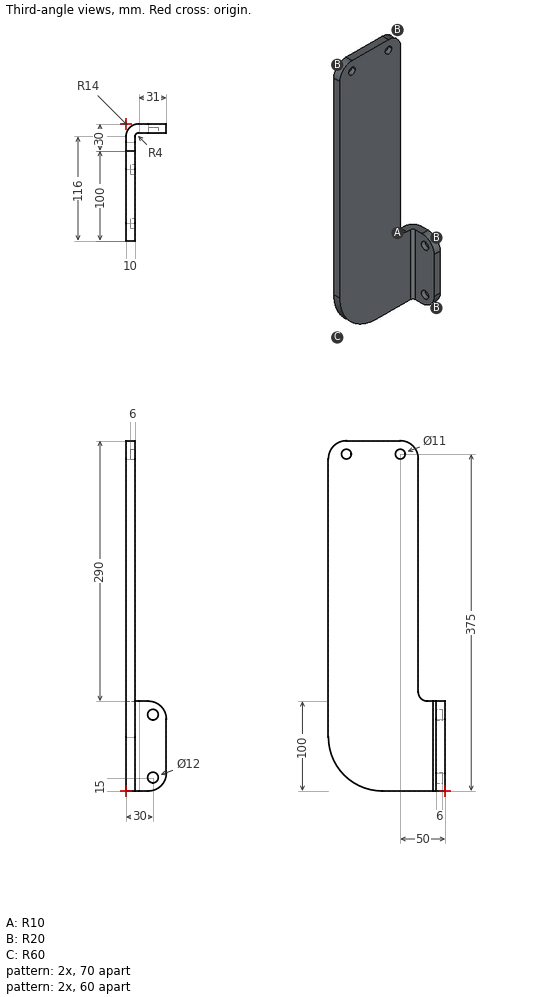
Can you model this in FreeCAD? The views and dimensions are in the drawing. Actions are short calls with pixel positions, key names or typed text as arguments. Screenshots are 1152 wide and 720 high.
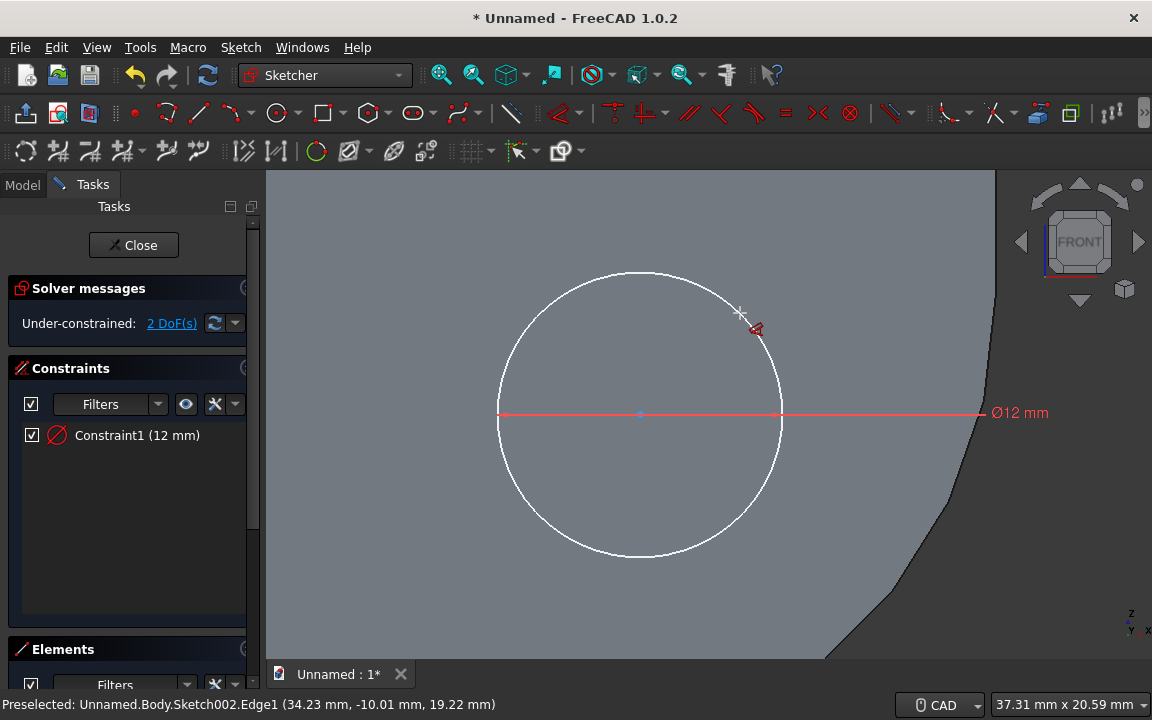
click(640, 415)
click(467, 381)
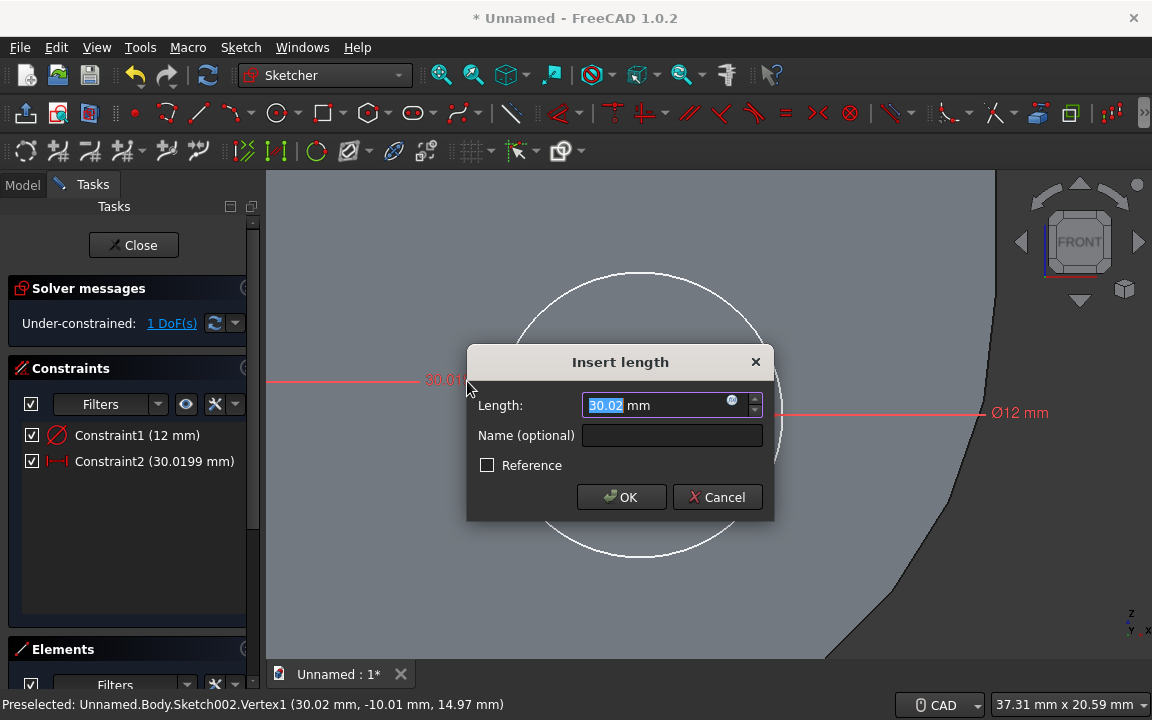
text(30)
key(Return)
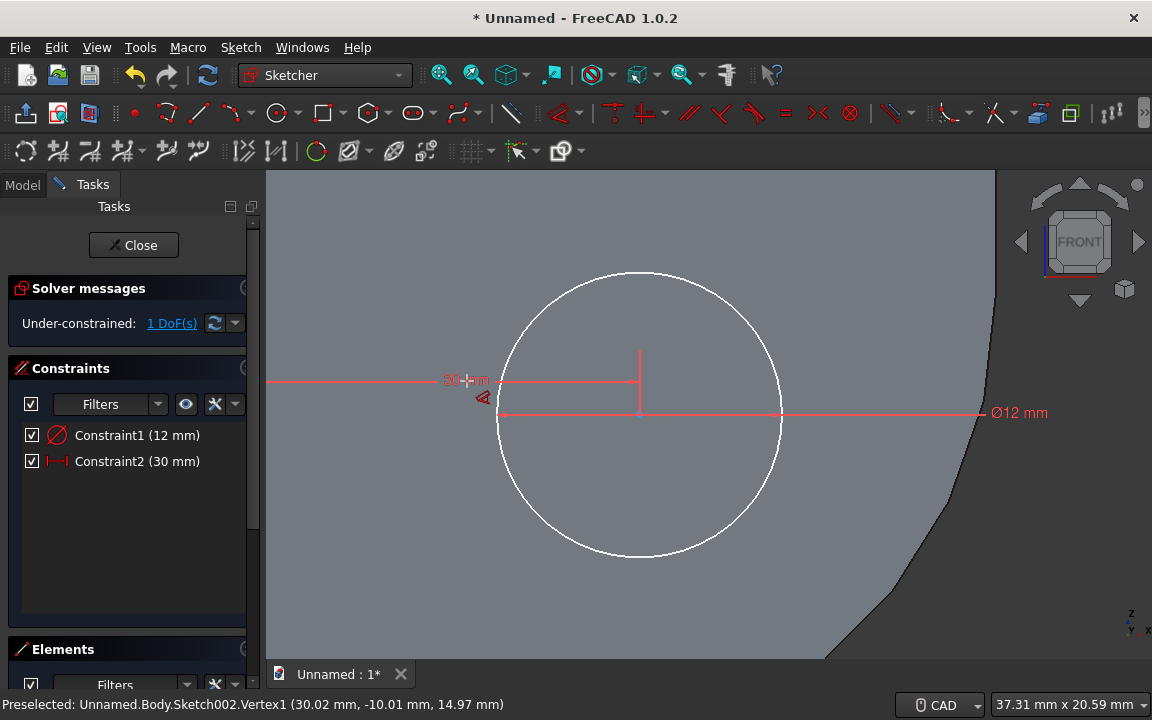
click(640, 415)
click(674, 523)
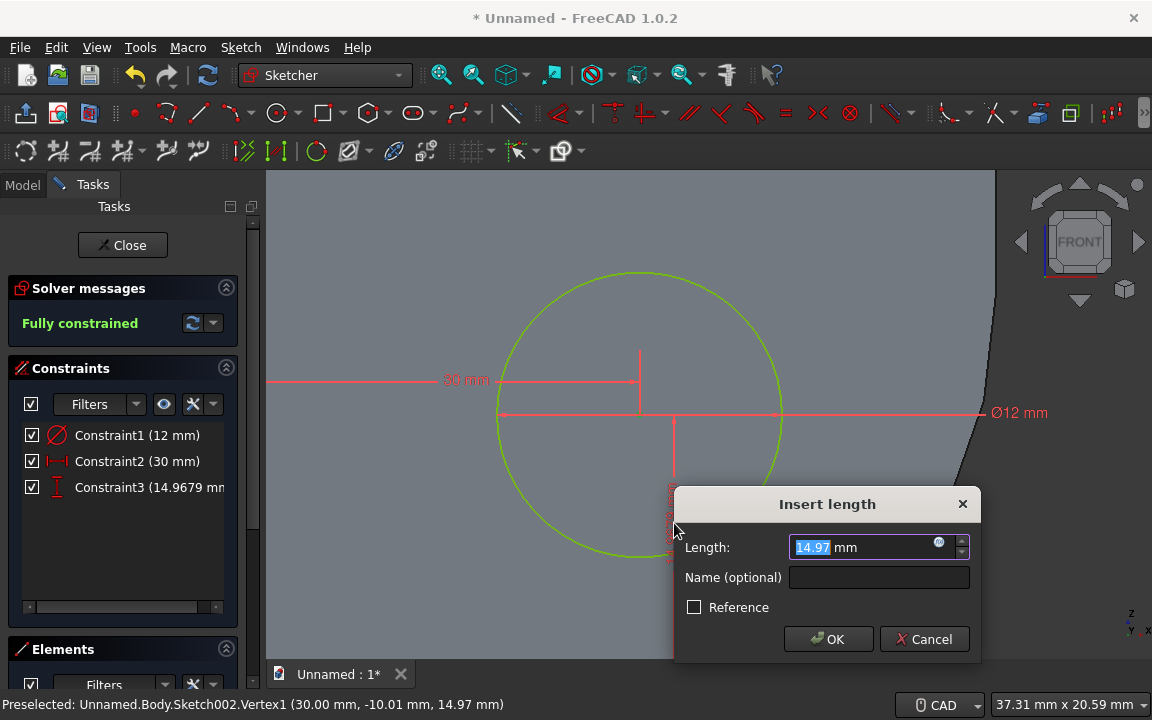
text(15)
key(Return)
key(Escape)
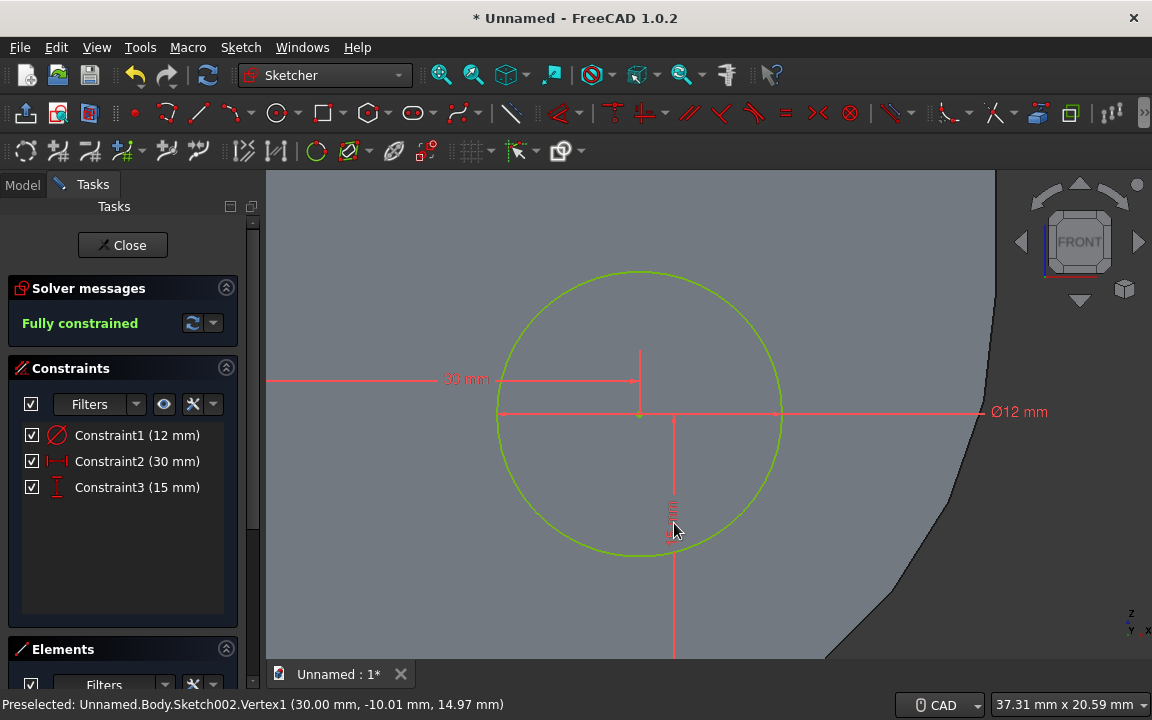
click(123, 245)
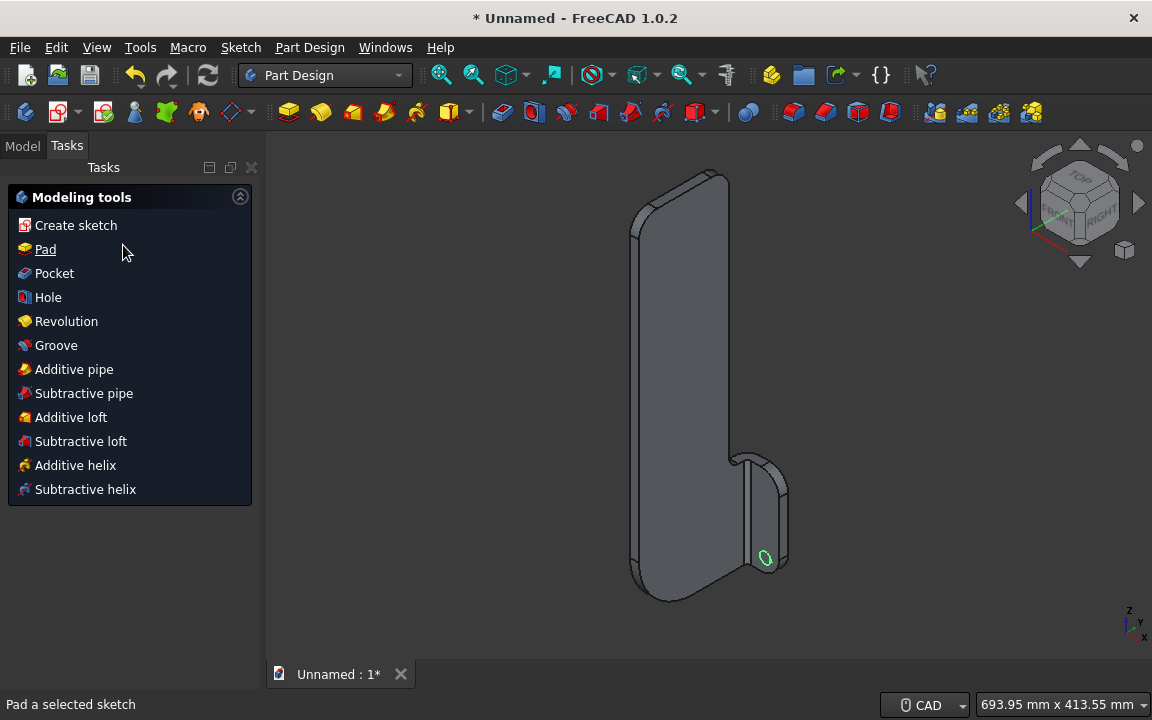
click(504, 112)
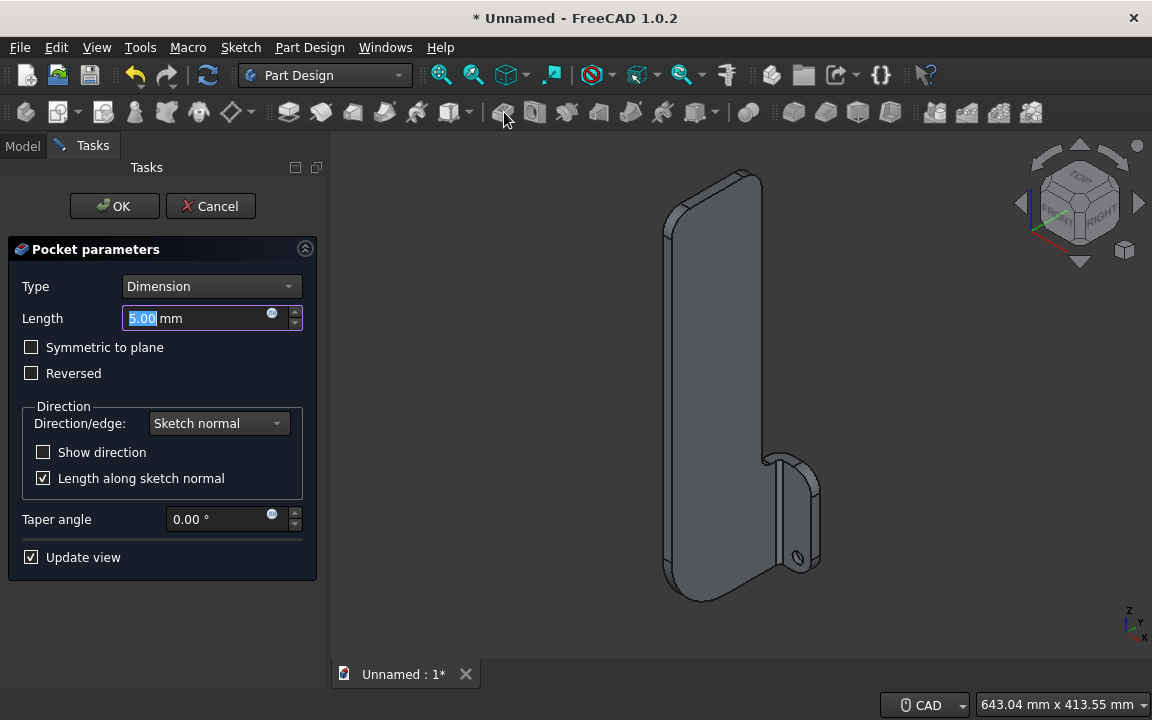
text(6)
key(Tab)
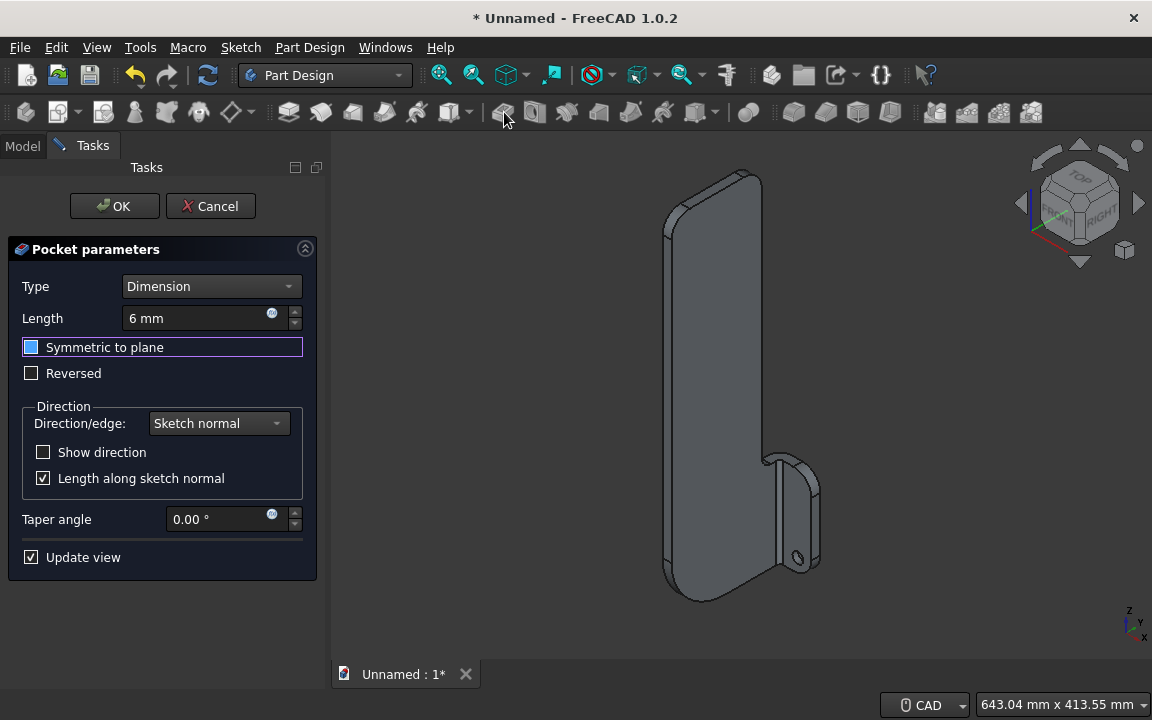
click(115, 206)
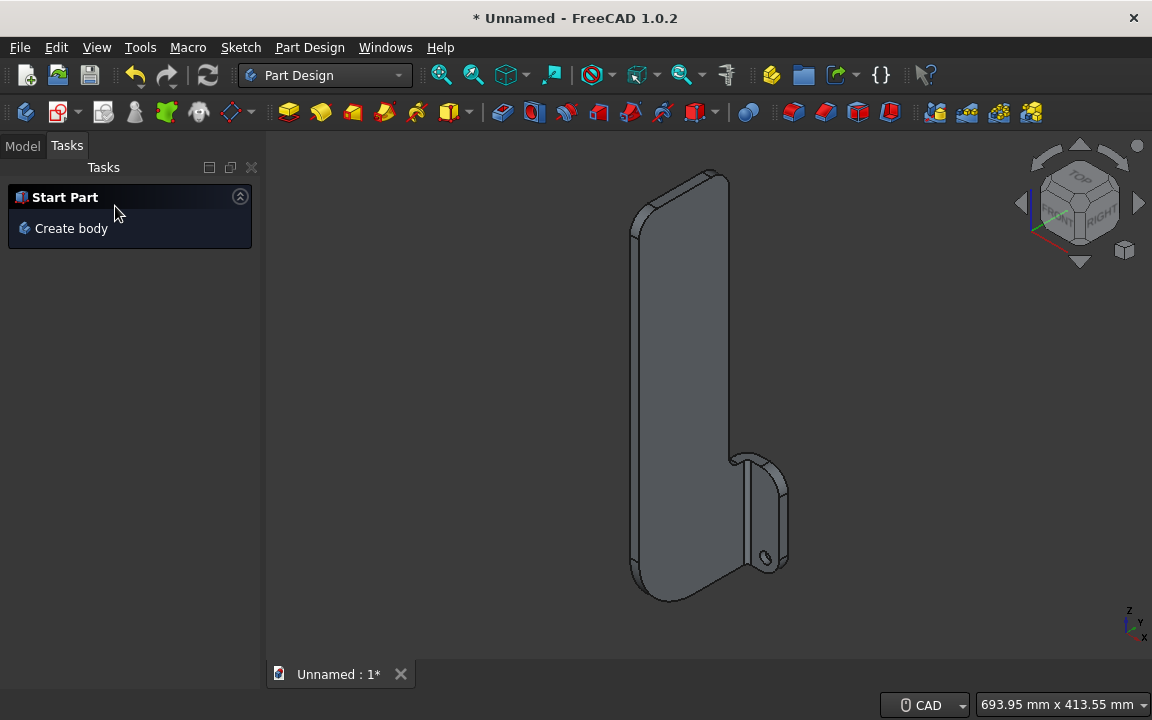
click(23, 145)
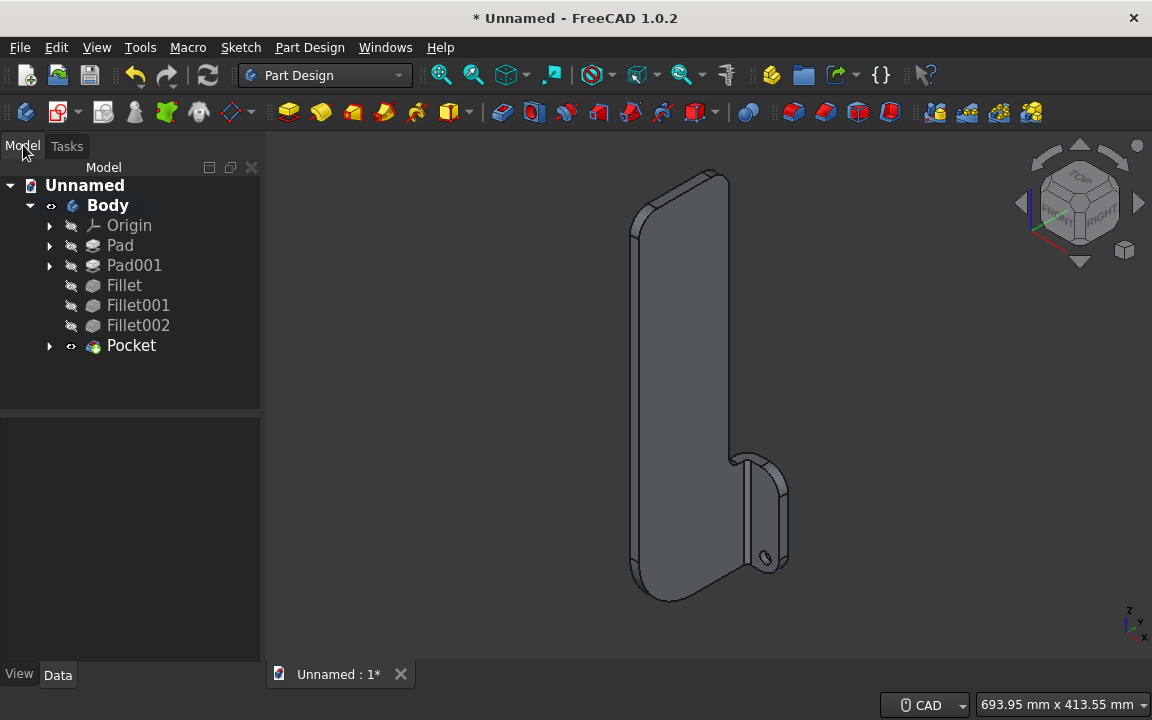
click(116, 346)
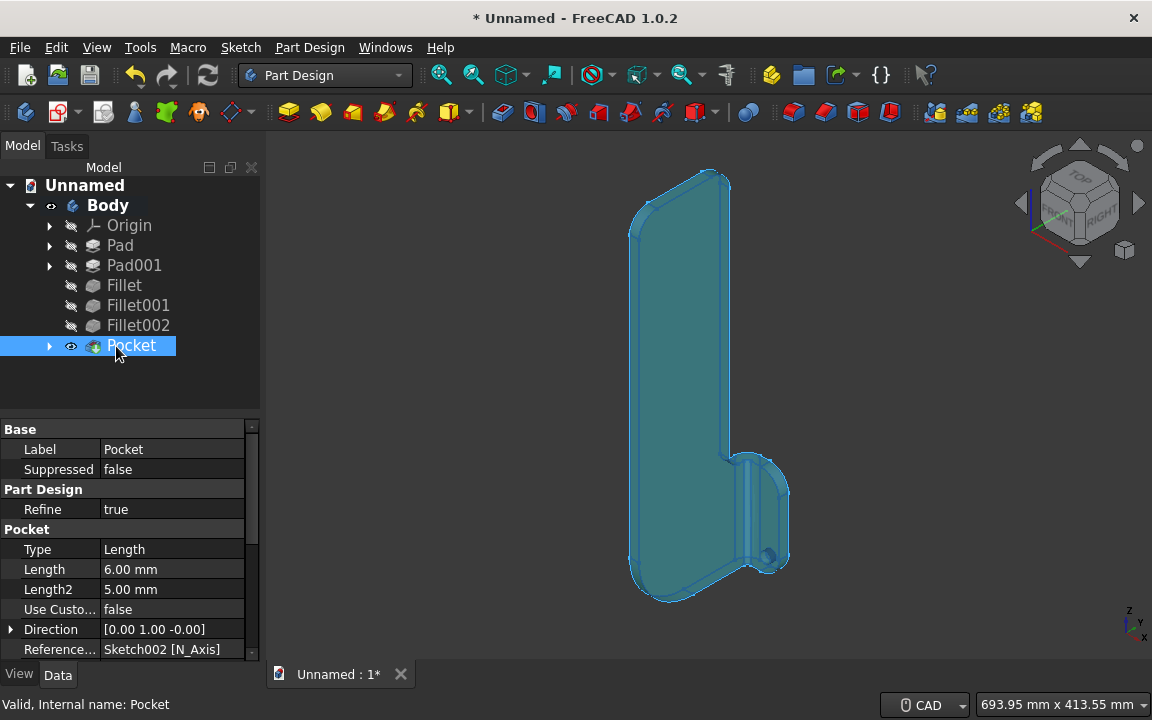
click(968, 112)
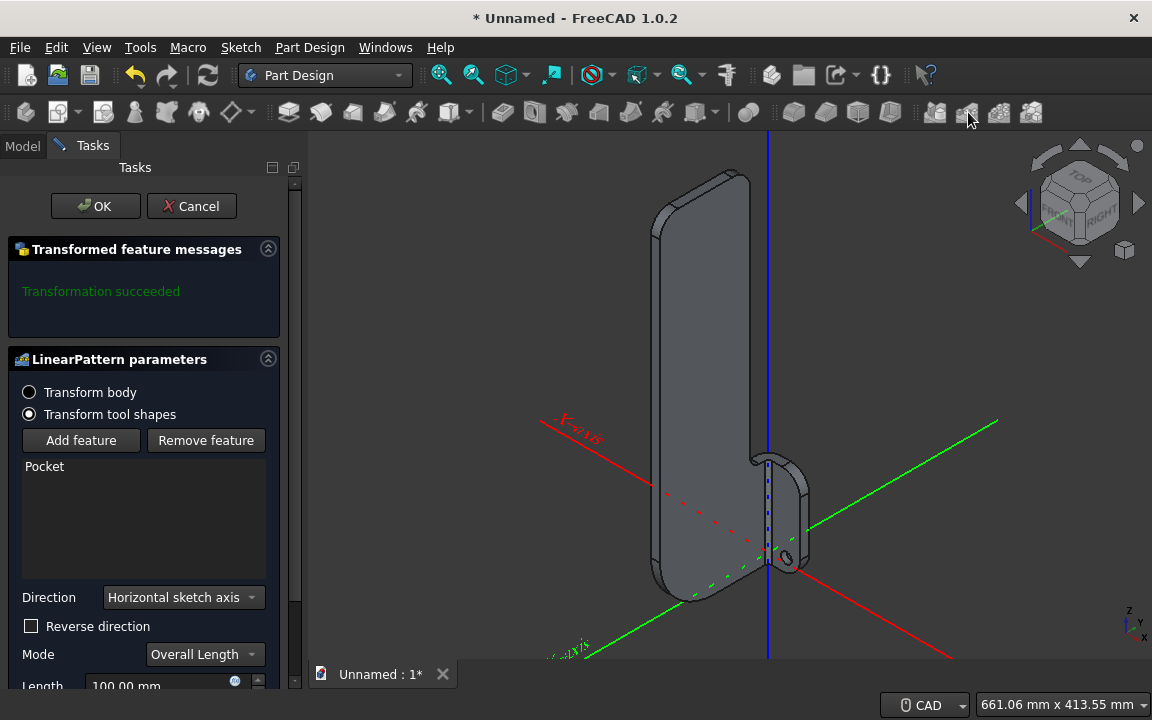
click(184, 598)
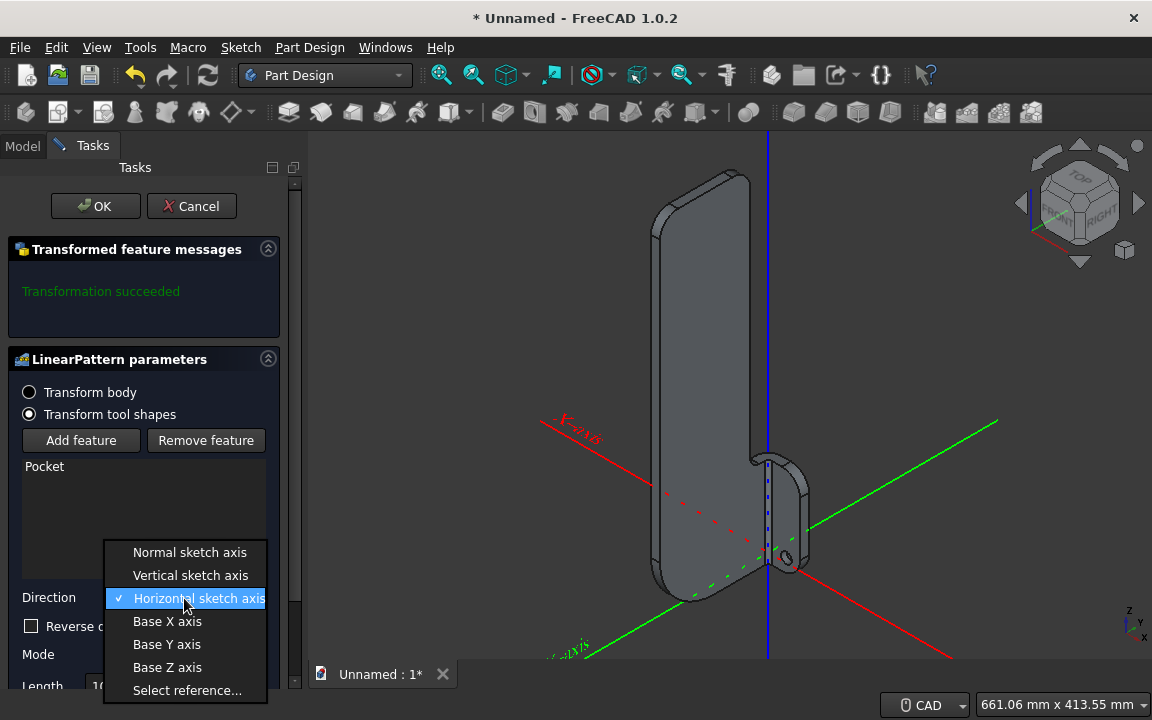
click(184, 668)